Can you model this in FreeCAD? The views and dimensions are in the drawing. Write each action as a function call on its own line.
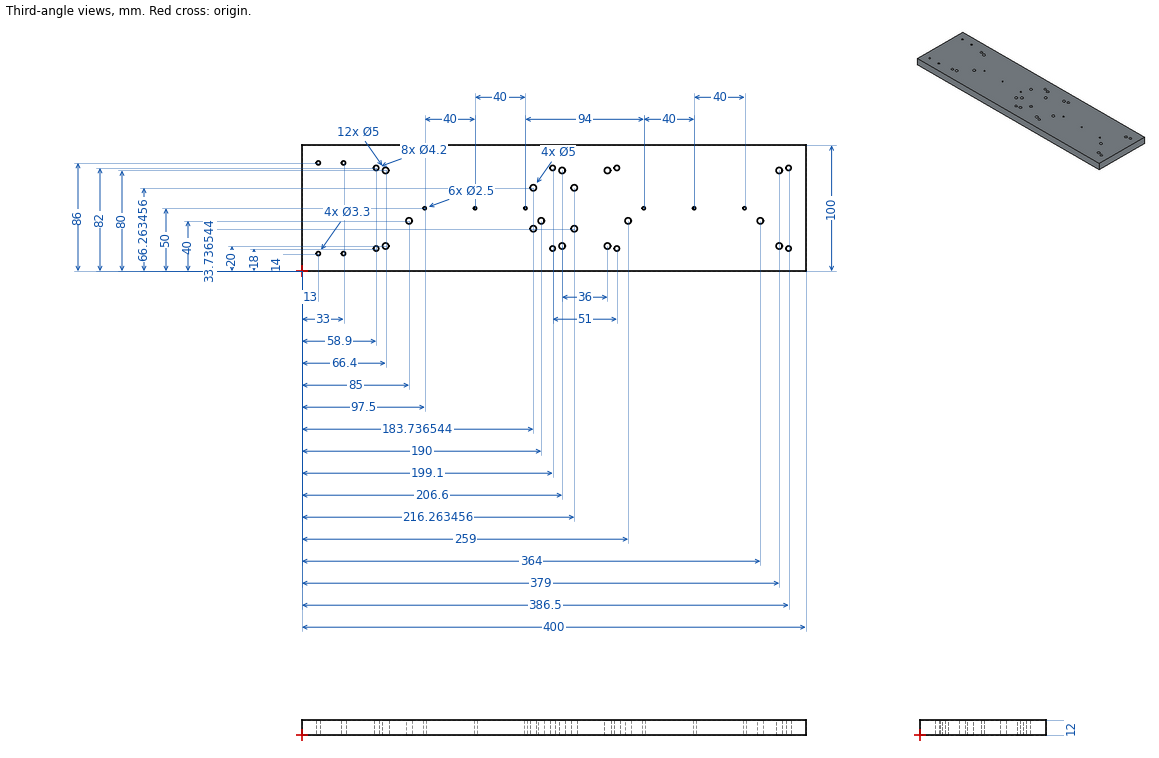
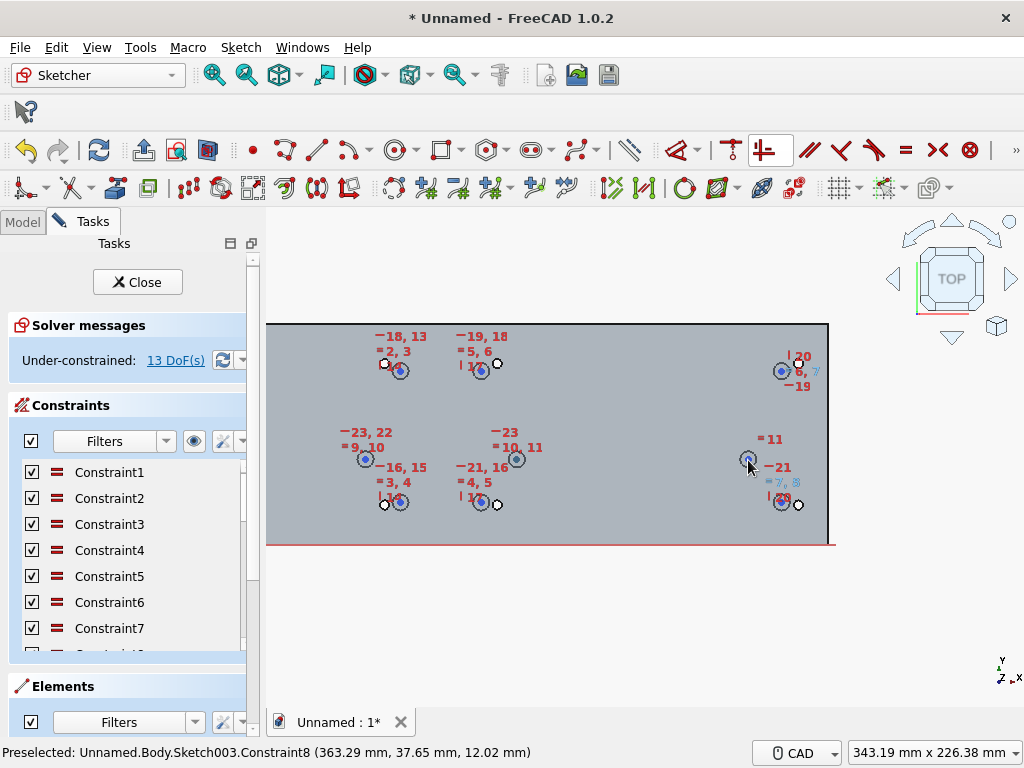
click(748, 459)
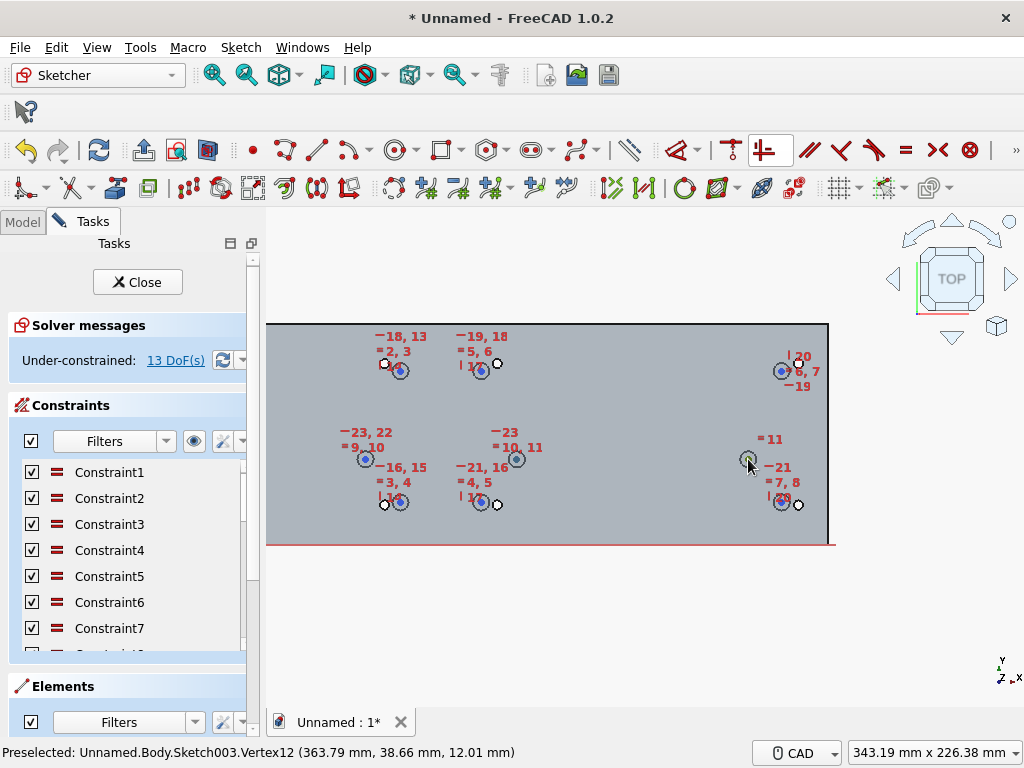
key(h)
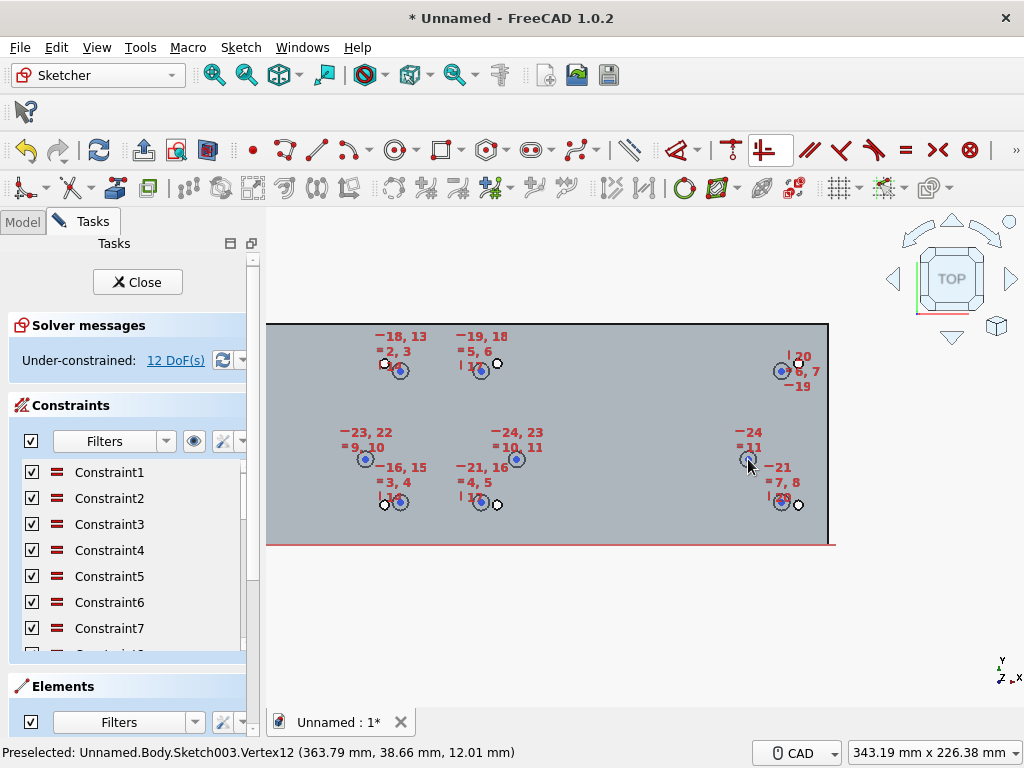
click(676, 150)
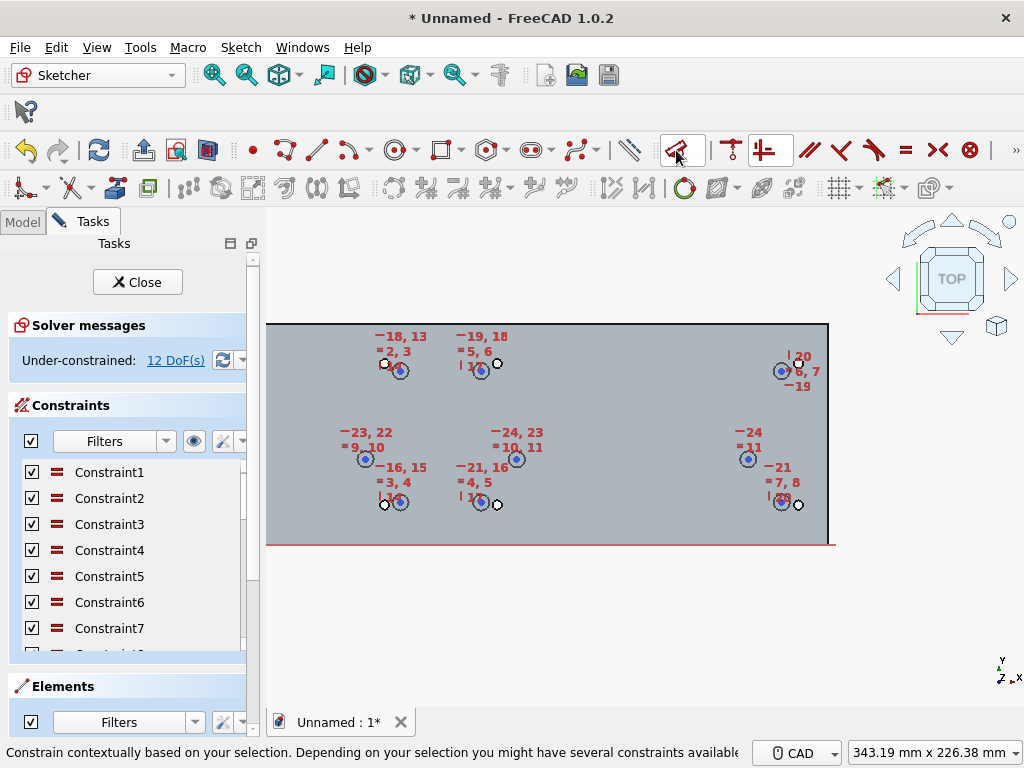
scroll(748, 460, down, 4)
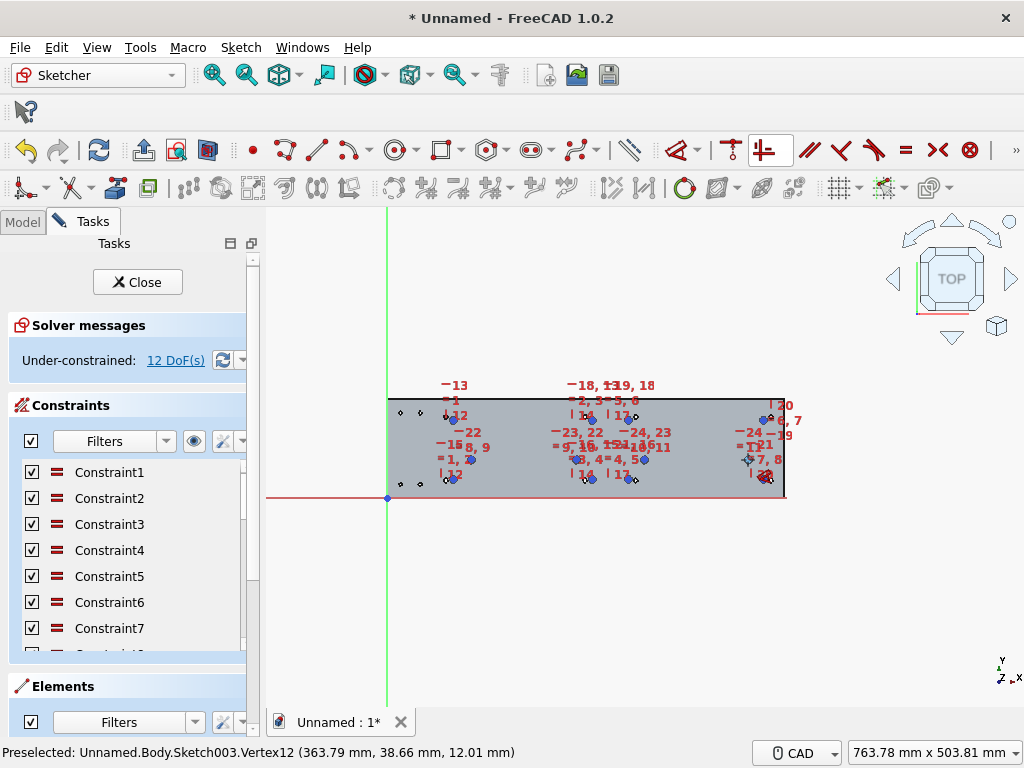
scroll(451, 423, up, 11)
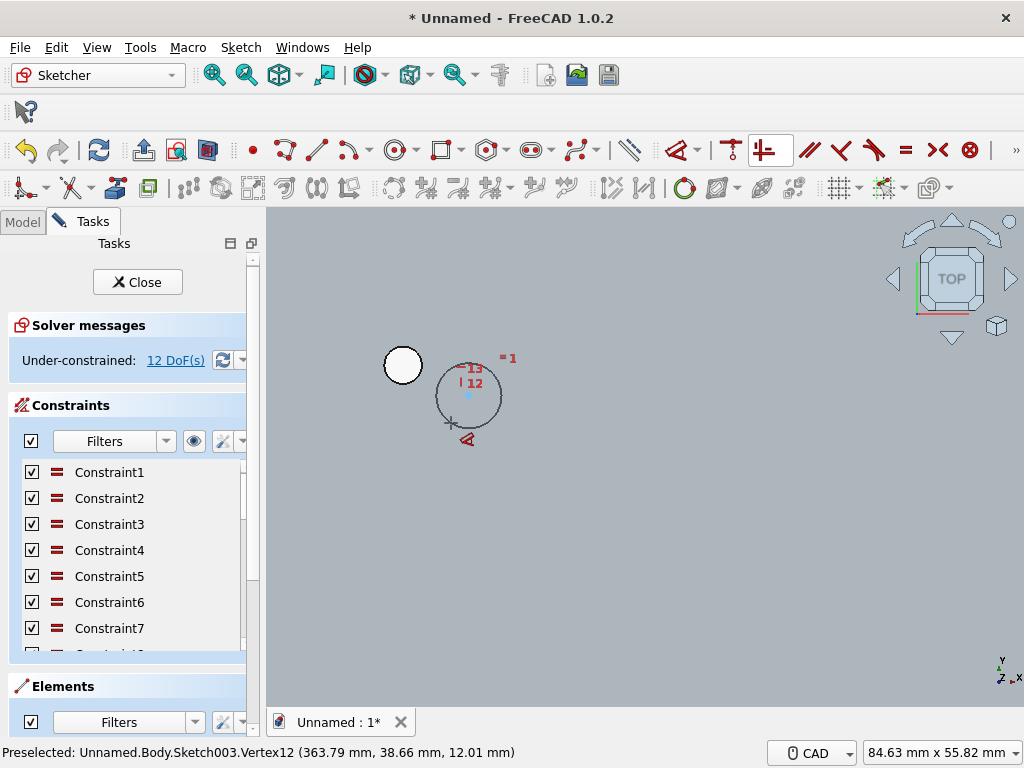
click(446, 419)
click(423, 442)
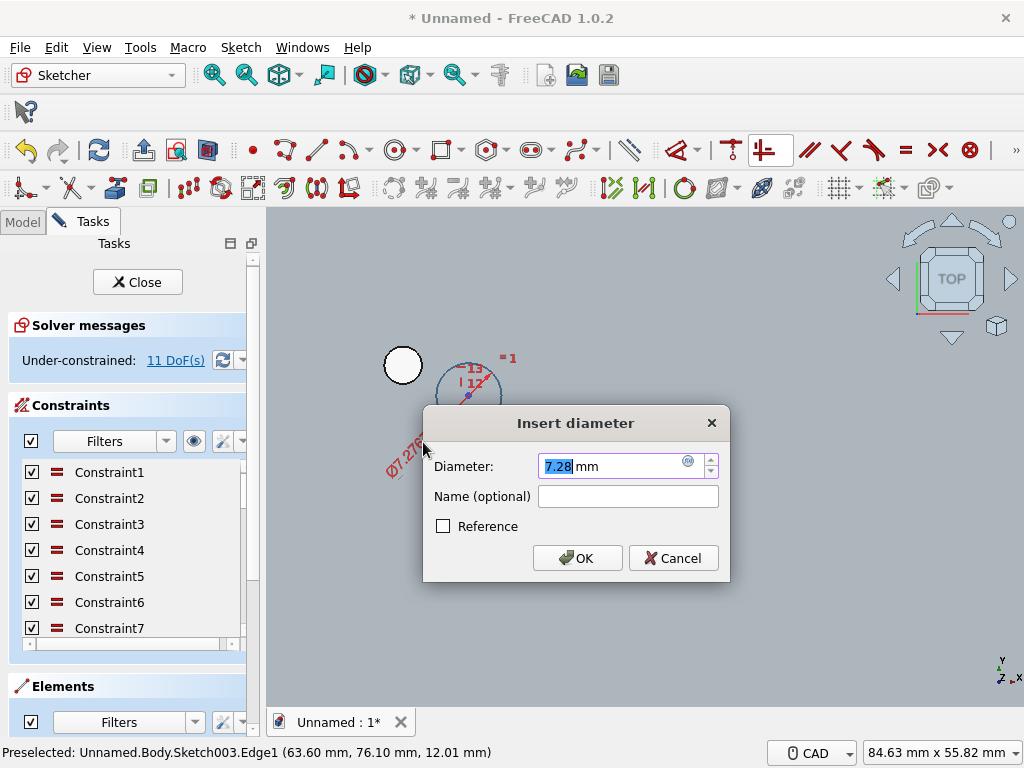
text(5)
key(Return)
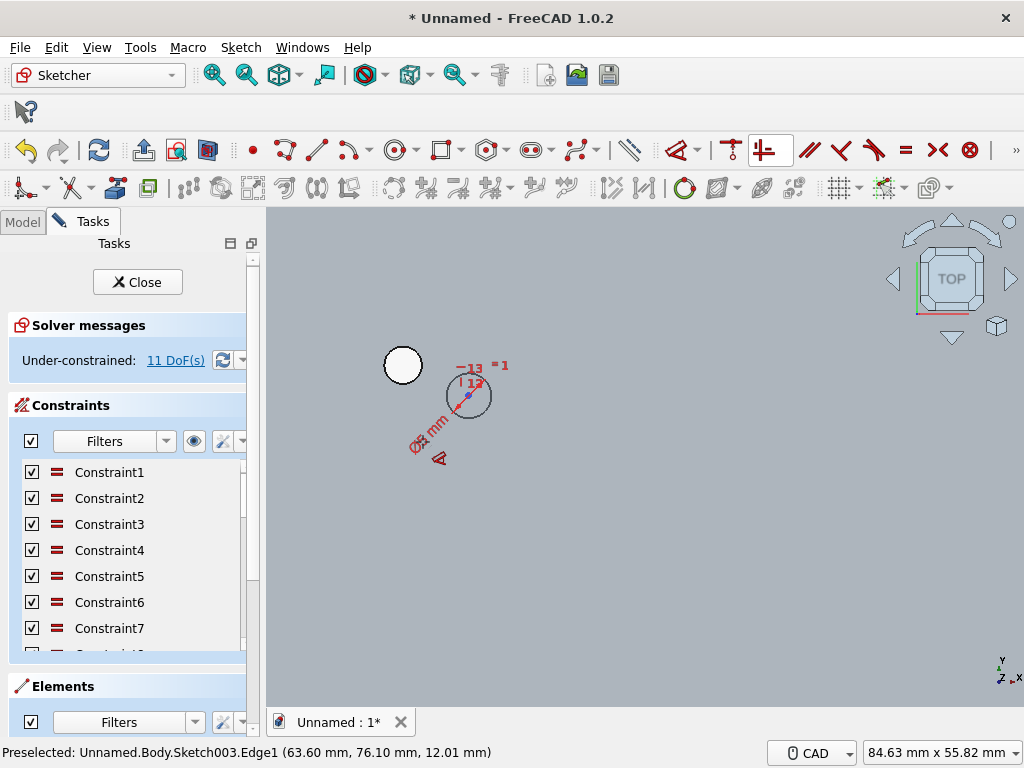
scroll(451, 423, down, 11)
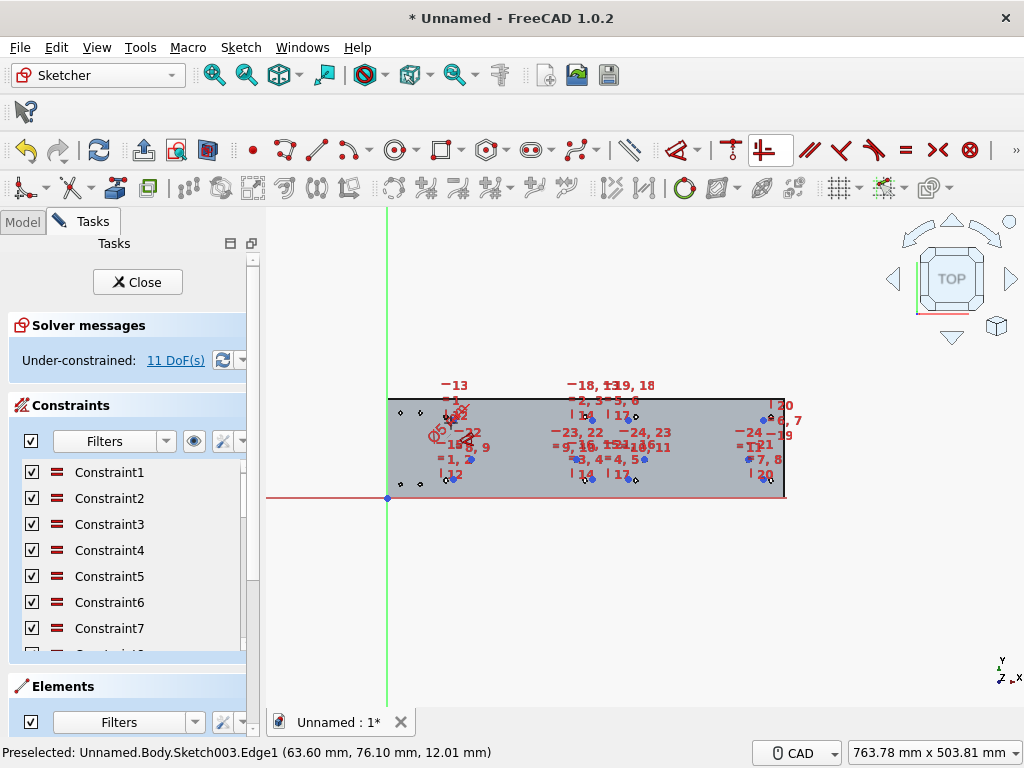
click(453, 420)
click(353, 459)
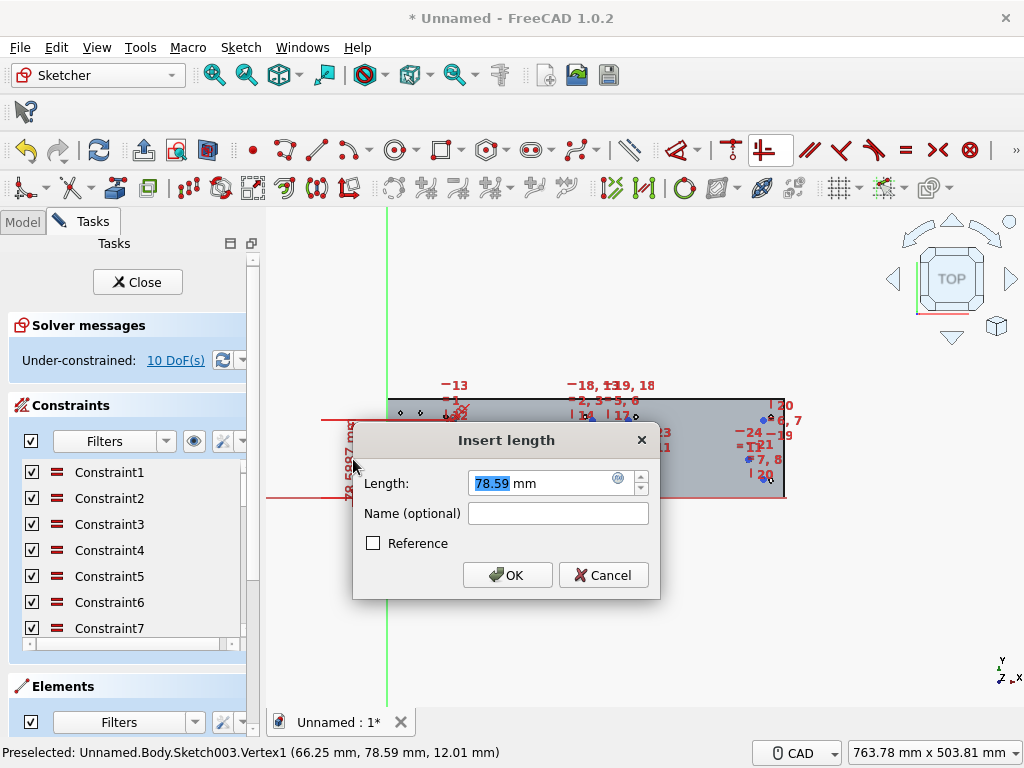
text(80)
key(Return)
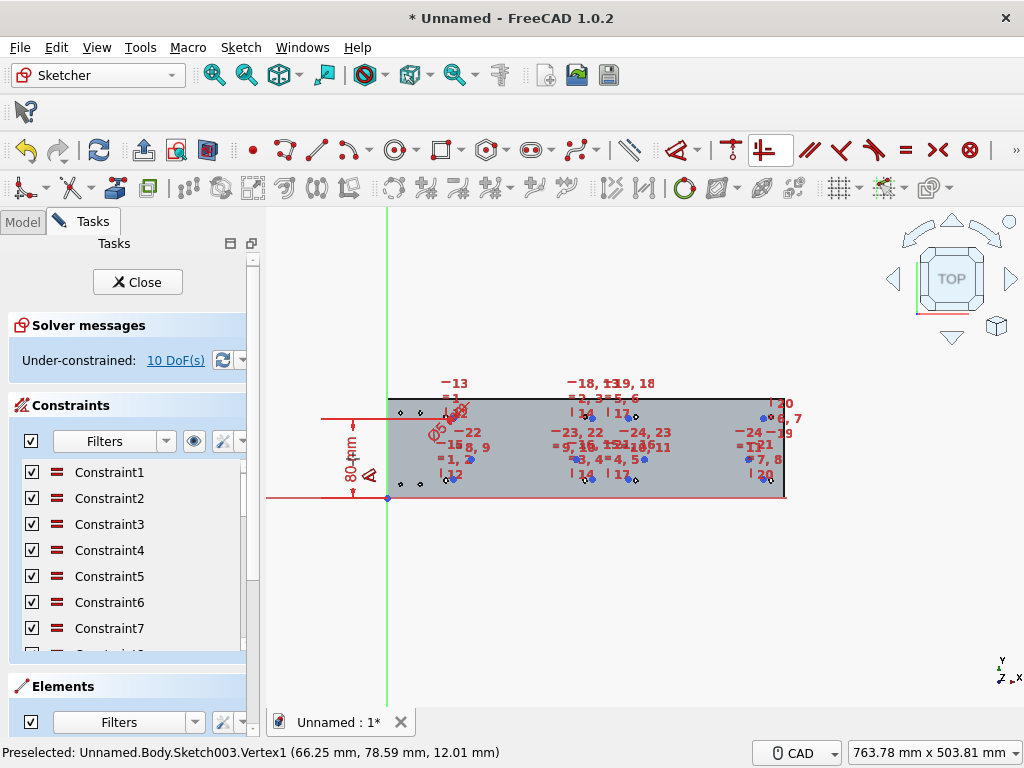
scroll(453, 479, up, 4)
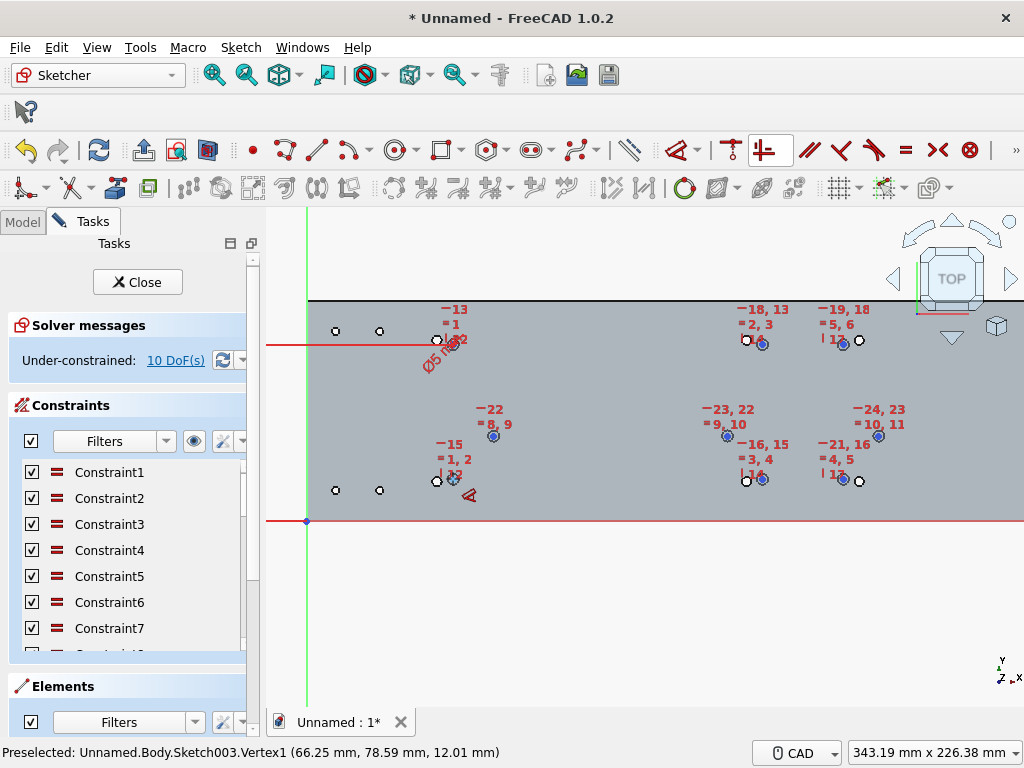
click(453, 479)
click(487, 500)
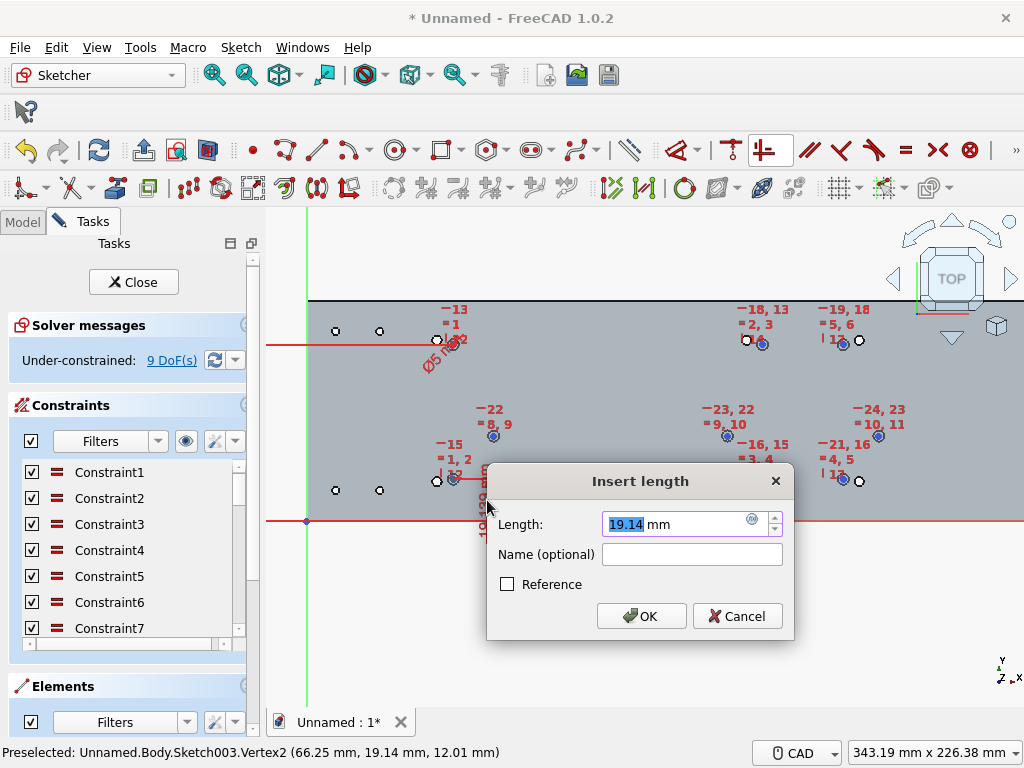
text(20)
key(Return)